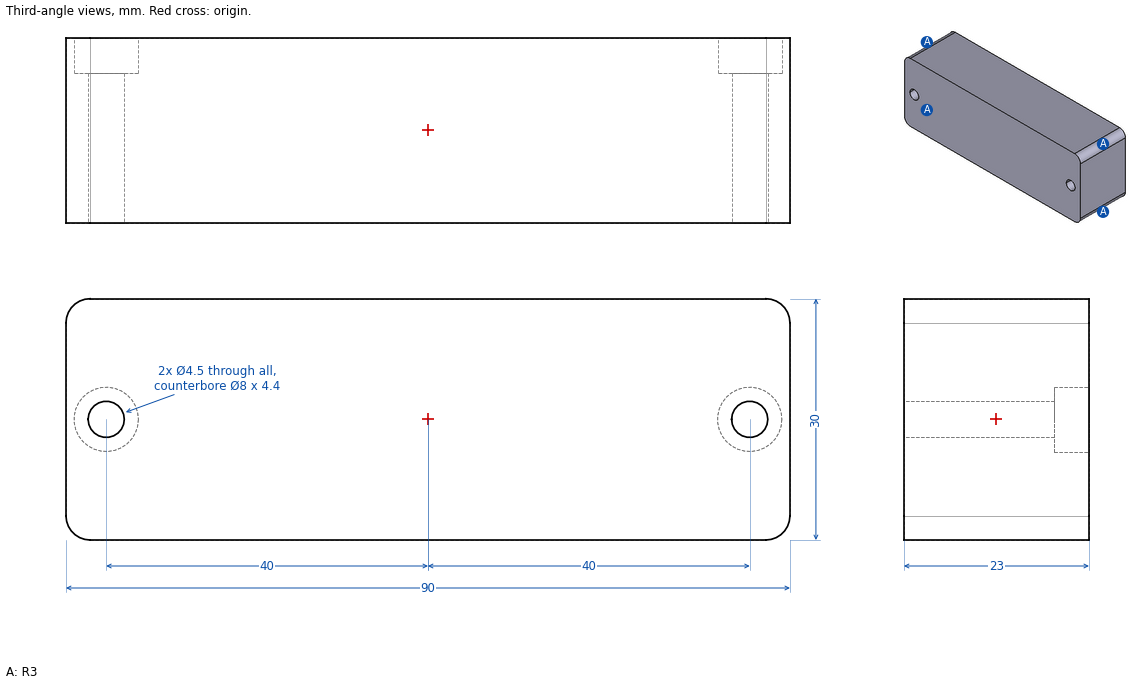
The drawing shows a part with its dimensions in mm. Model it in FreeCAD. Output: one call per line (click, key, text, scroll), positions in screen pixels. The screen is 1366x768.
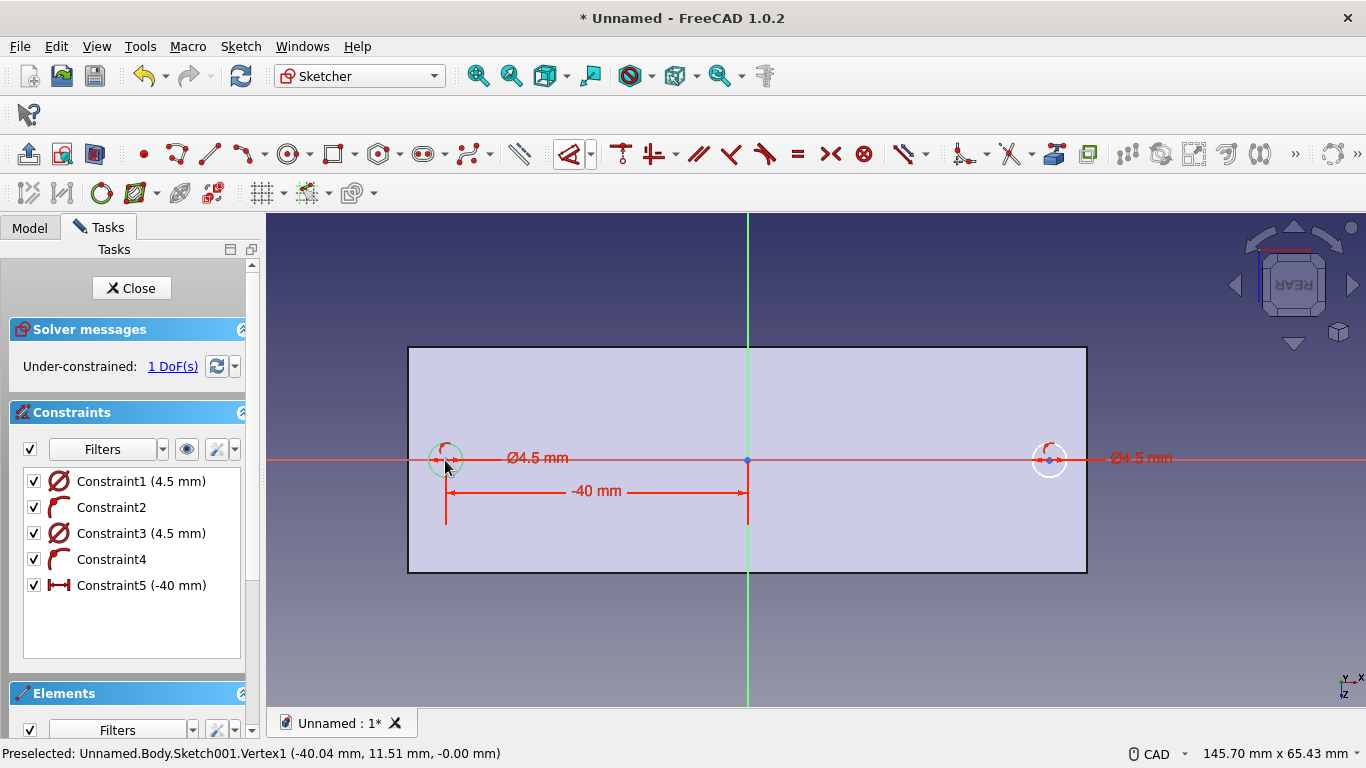
click(1050, 460)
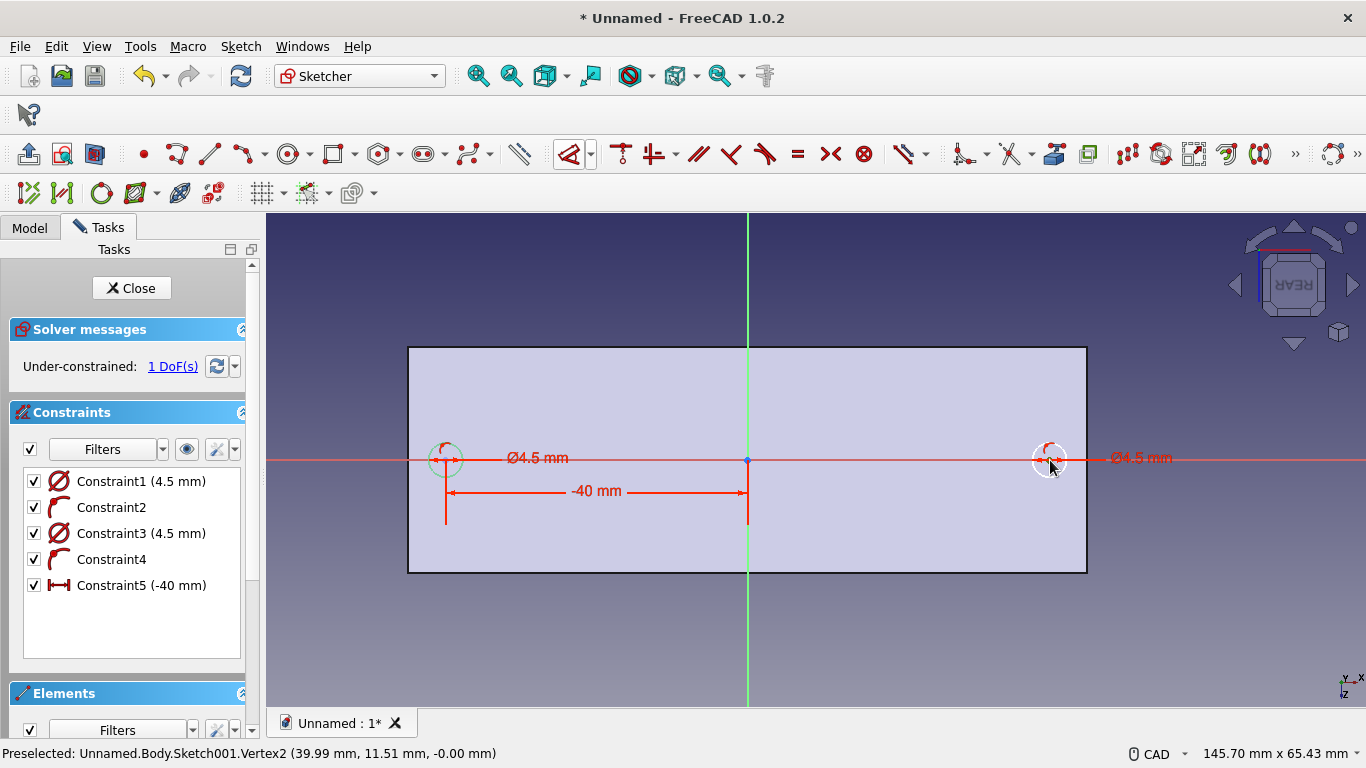
key(l)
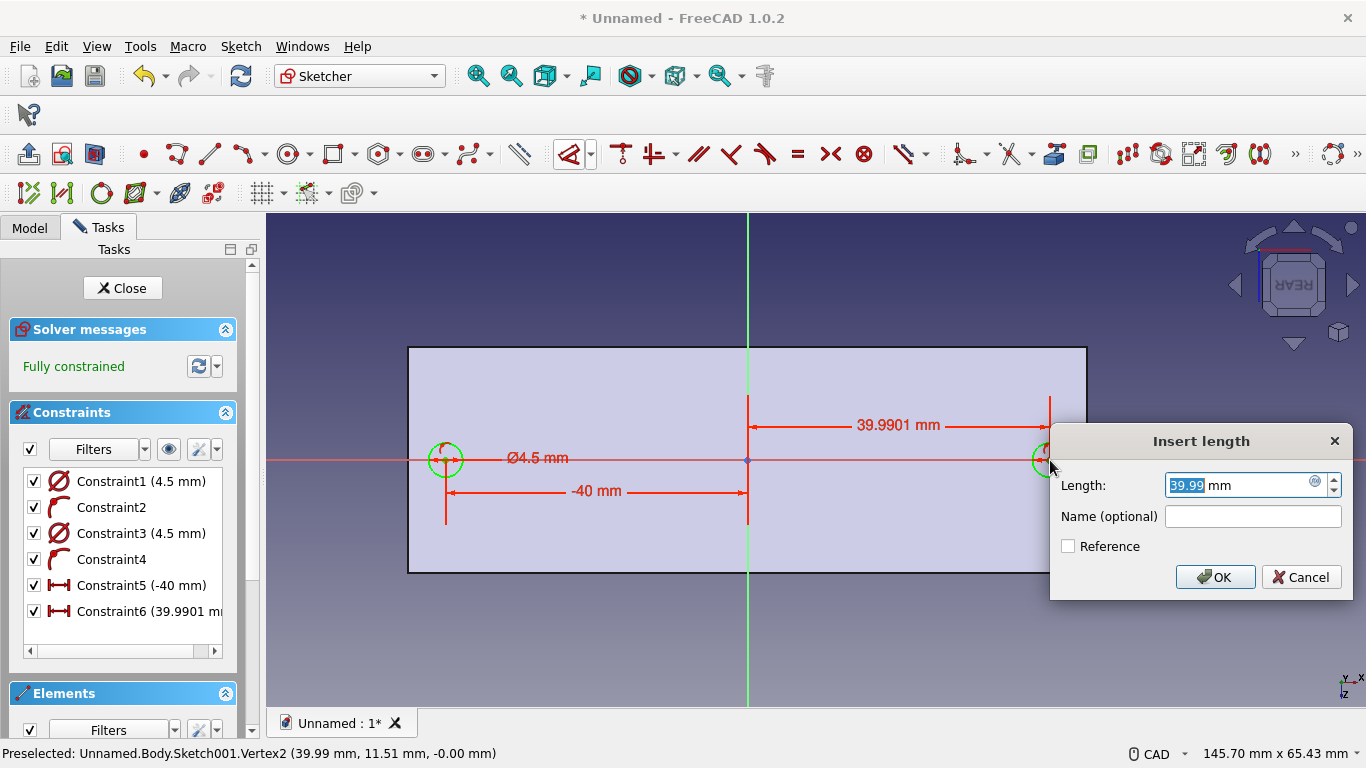
text(40)
key(Return)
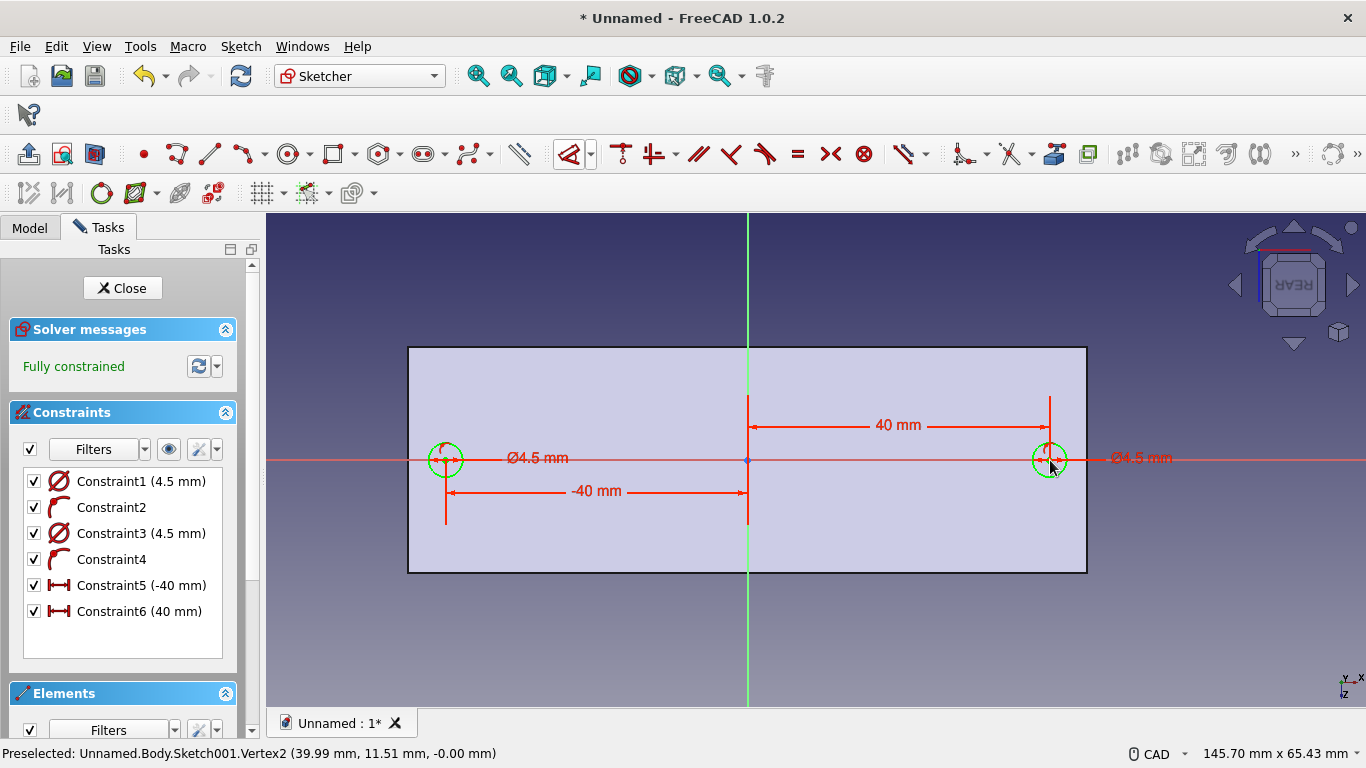
click(123, 288)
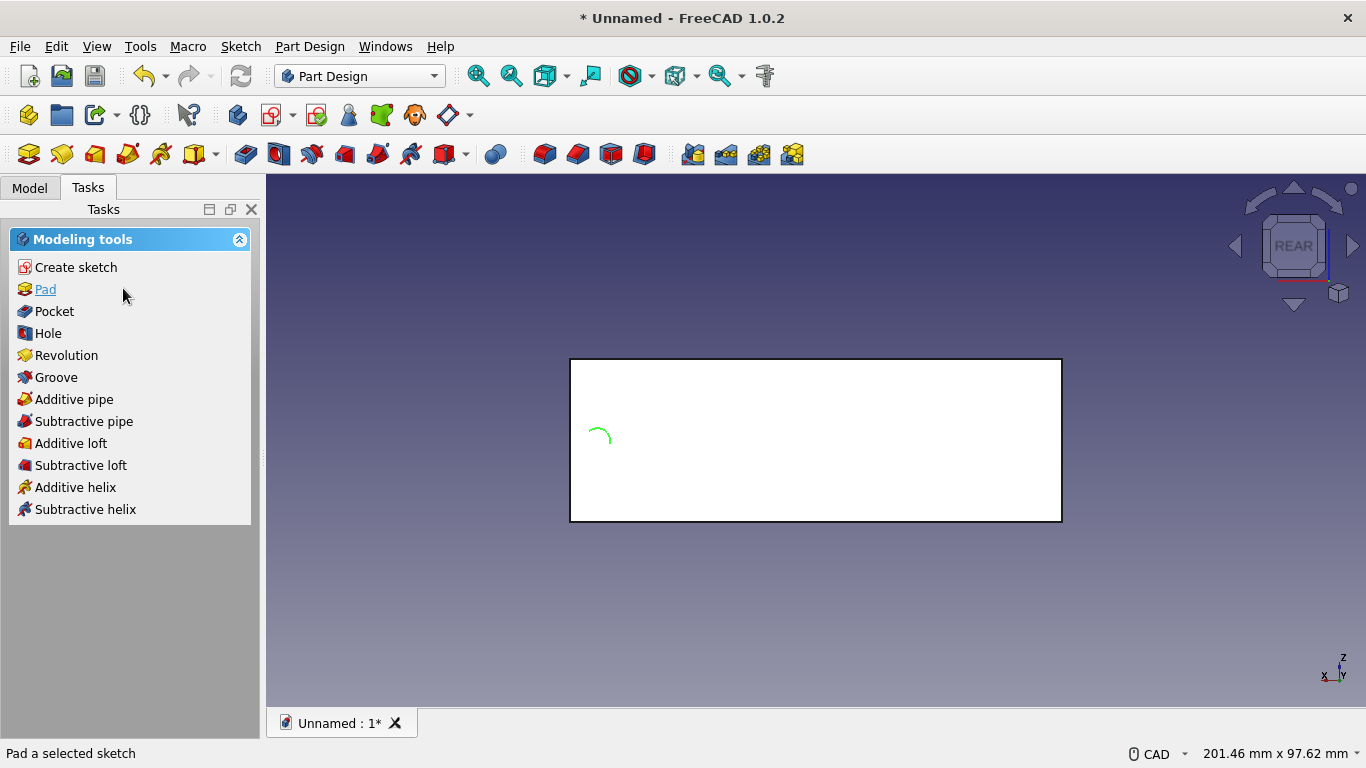
click(279, 154)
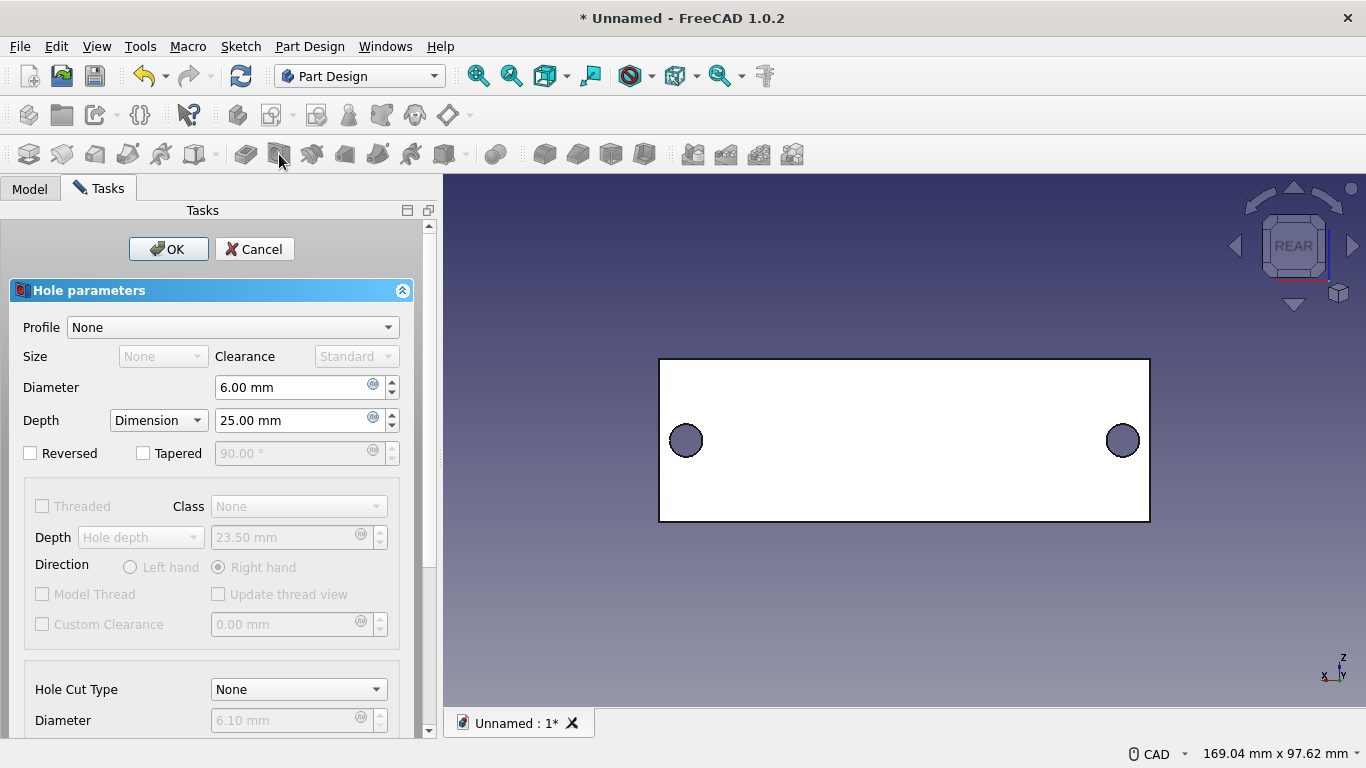
triple_click(300, 388)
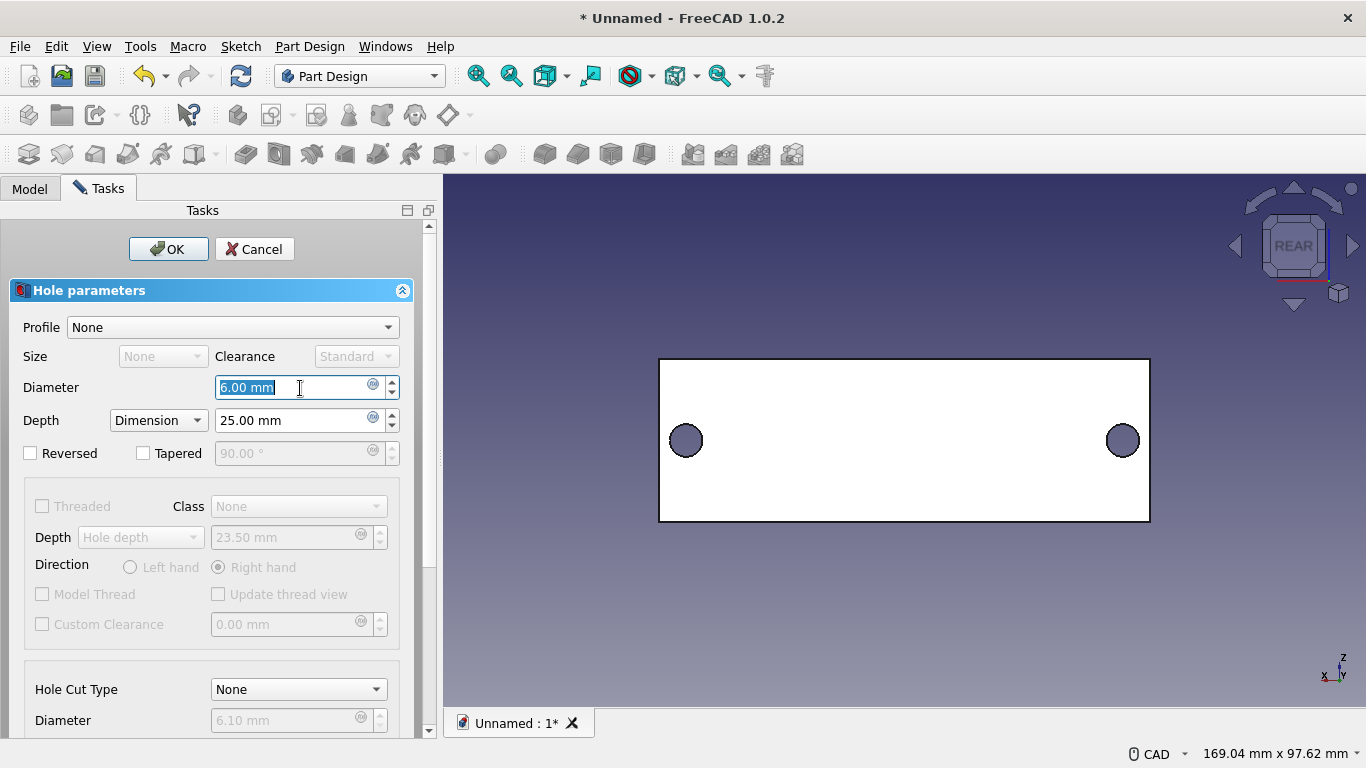
text(4.5)
key(Tab)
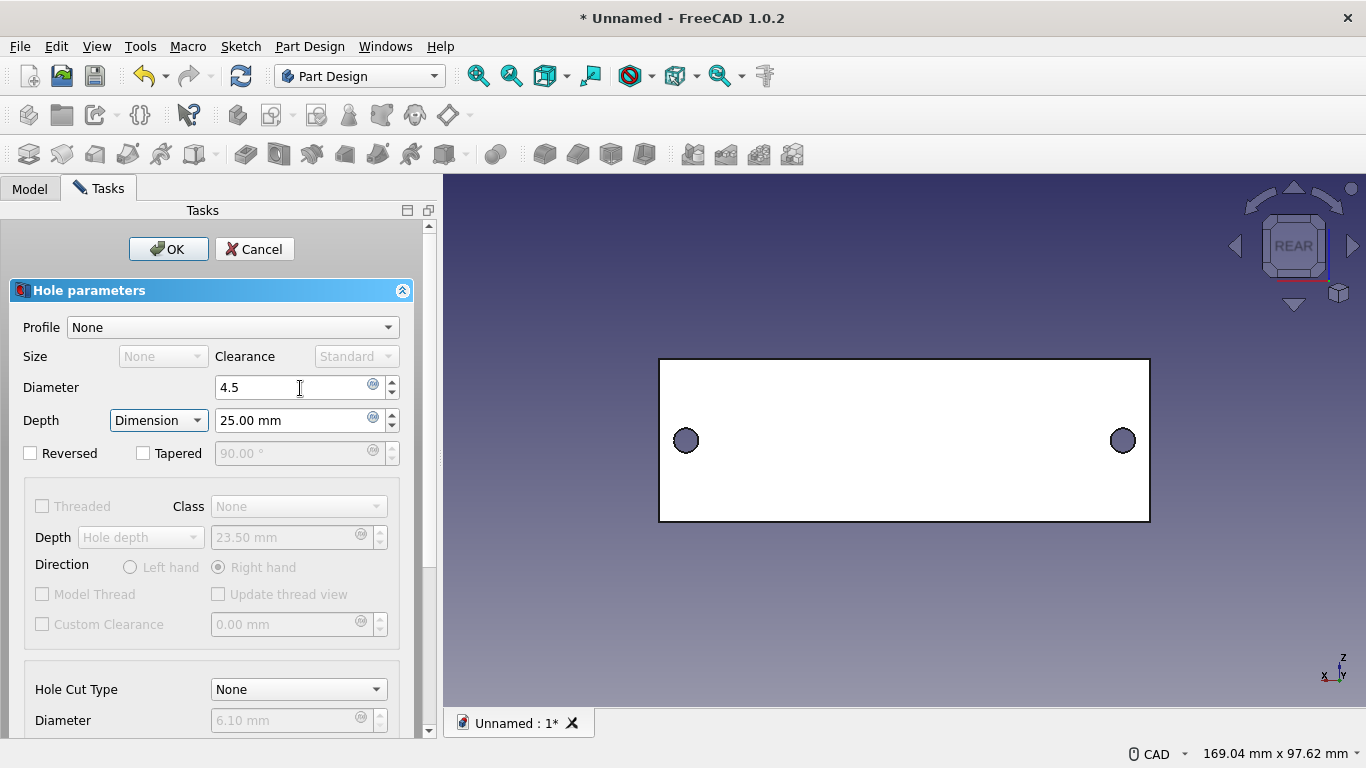
click(160, 420)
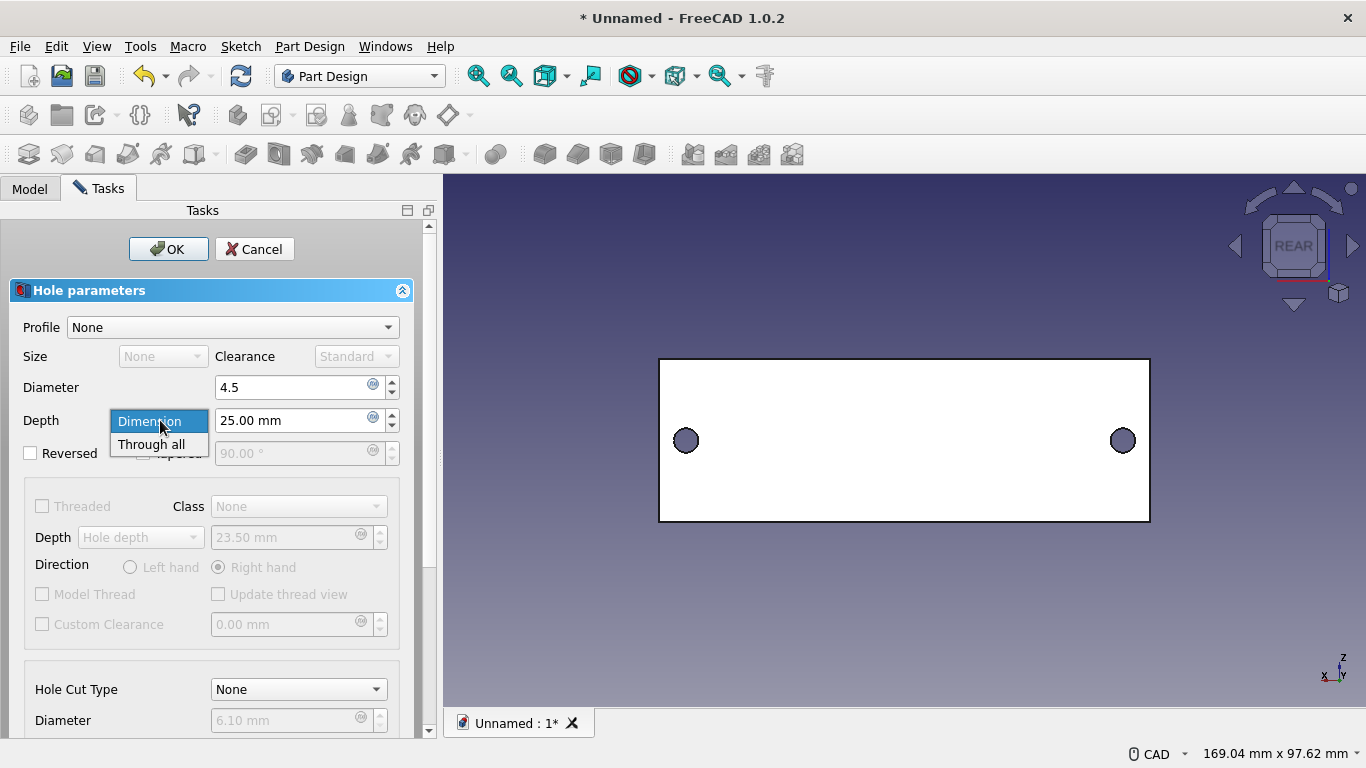
click(158, 444)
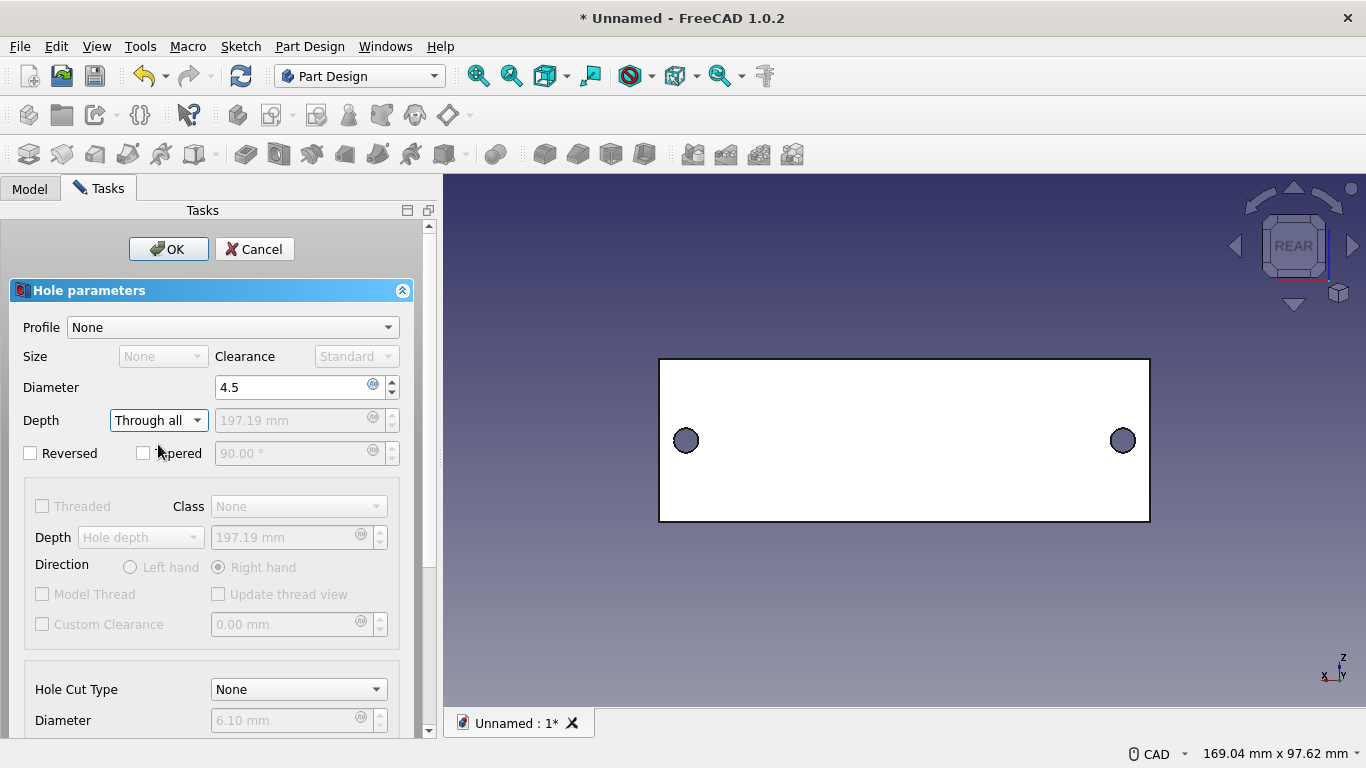
click(300, 690)